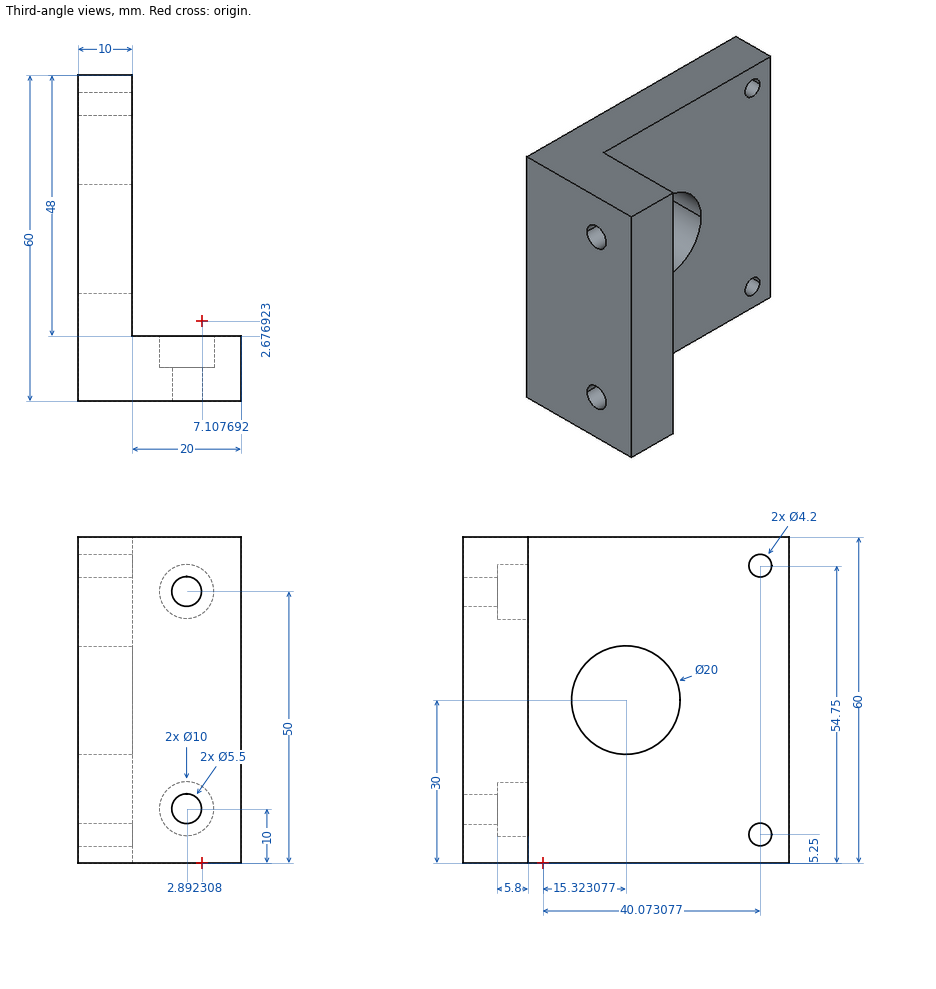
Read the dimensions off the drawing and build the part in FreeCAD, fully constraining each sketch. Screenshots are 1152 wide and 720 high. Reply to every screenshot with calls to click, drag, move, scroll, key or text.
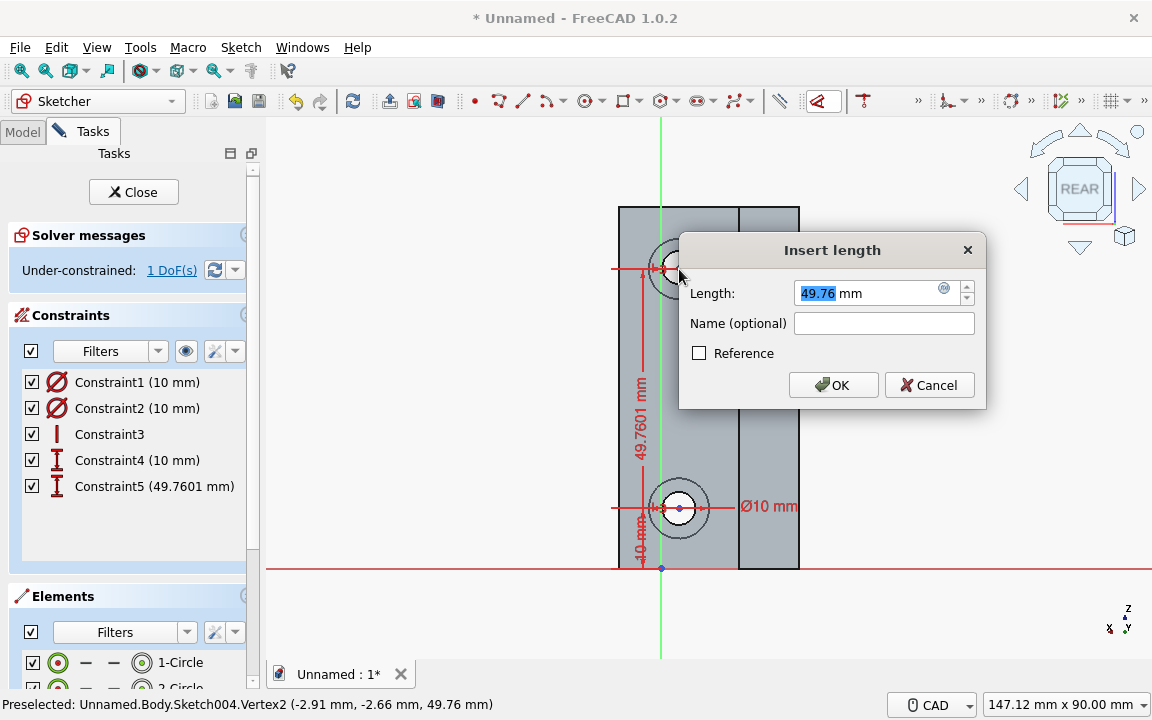
text(50)
key(Return)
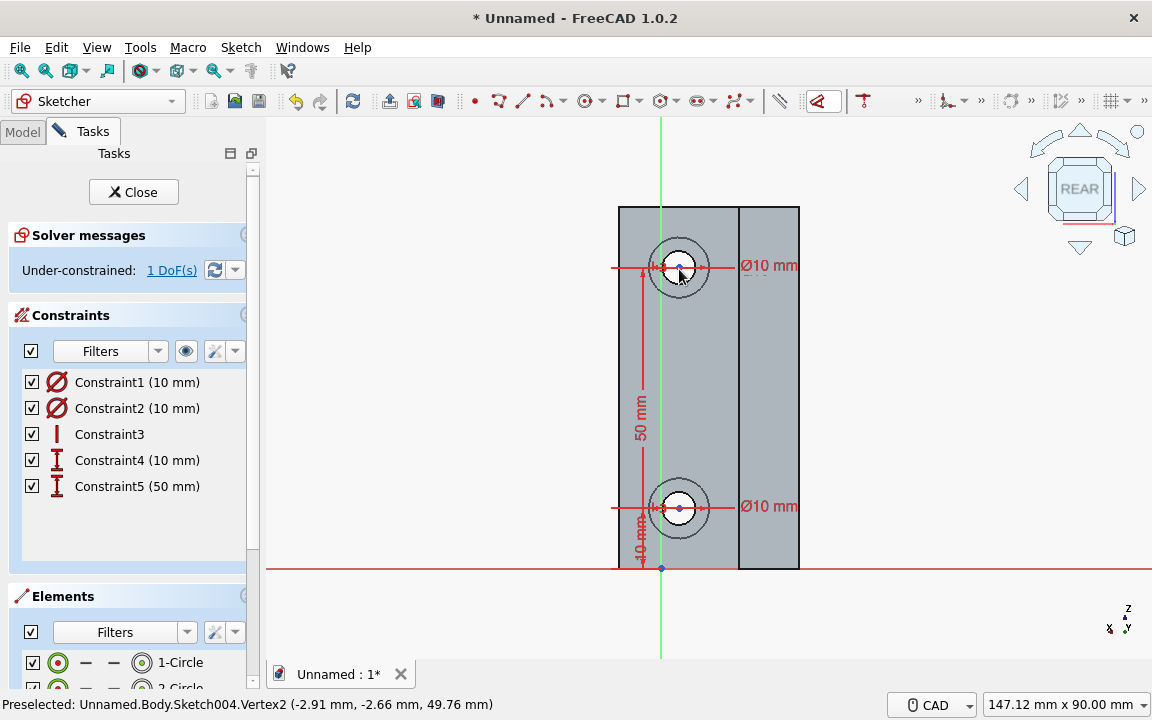
scroll(679, 508, up, 5)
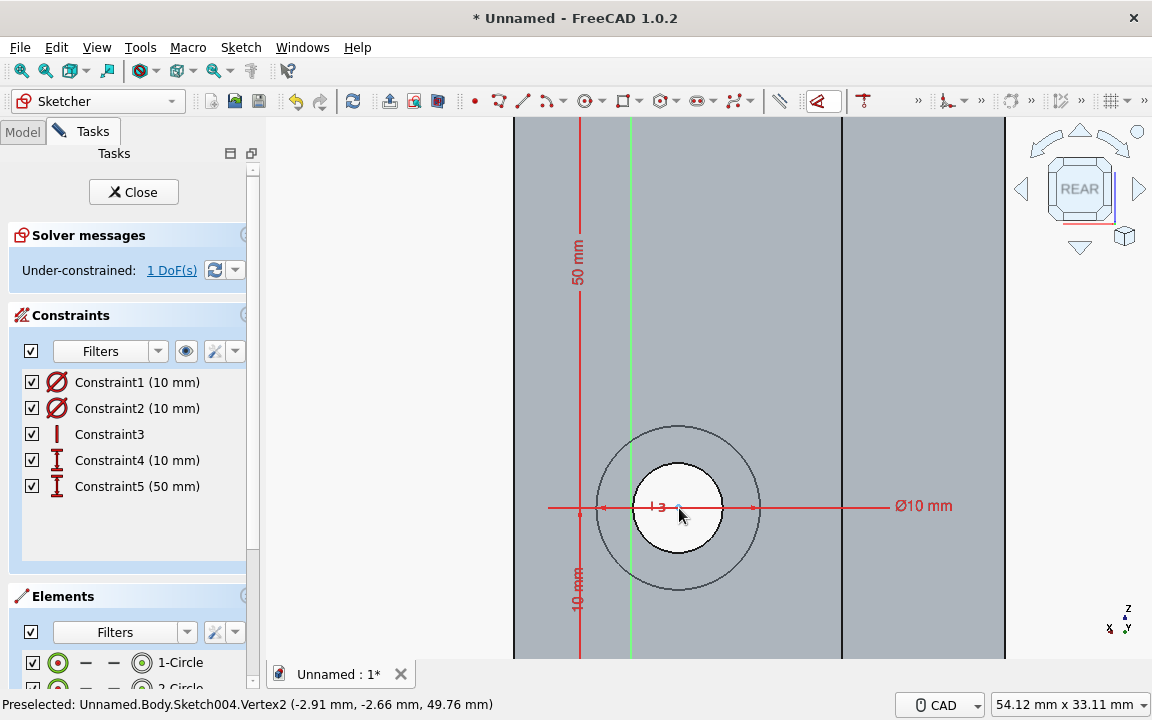
click(678, 508)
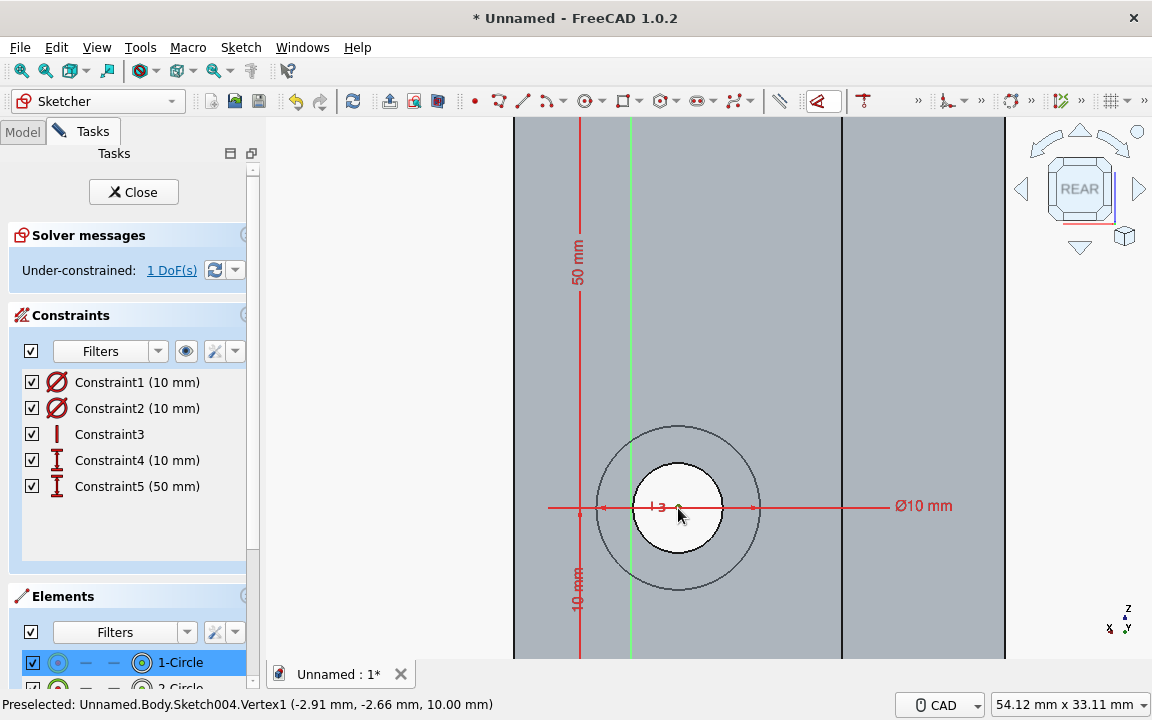
key(l)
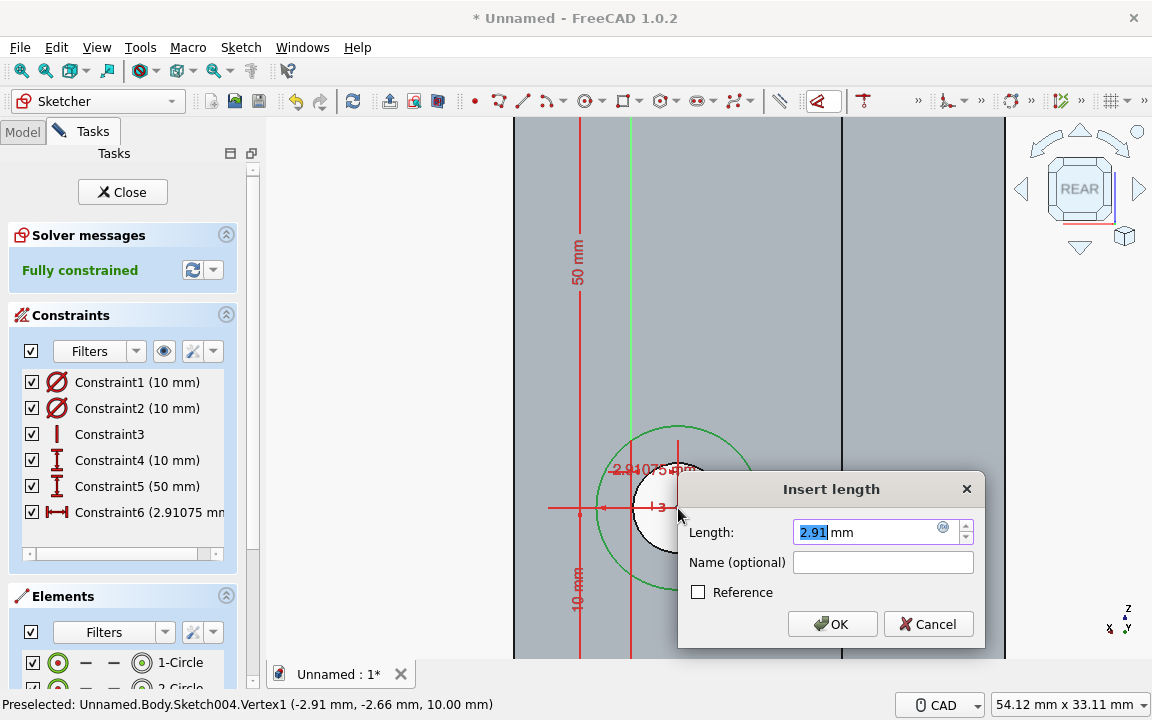
text(2.892308)
key(Return)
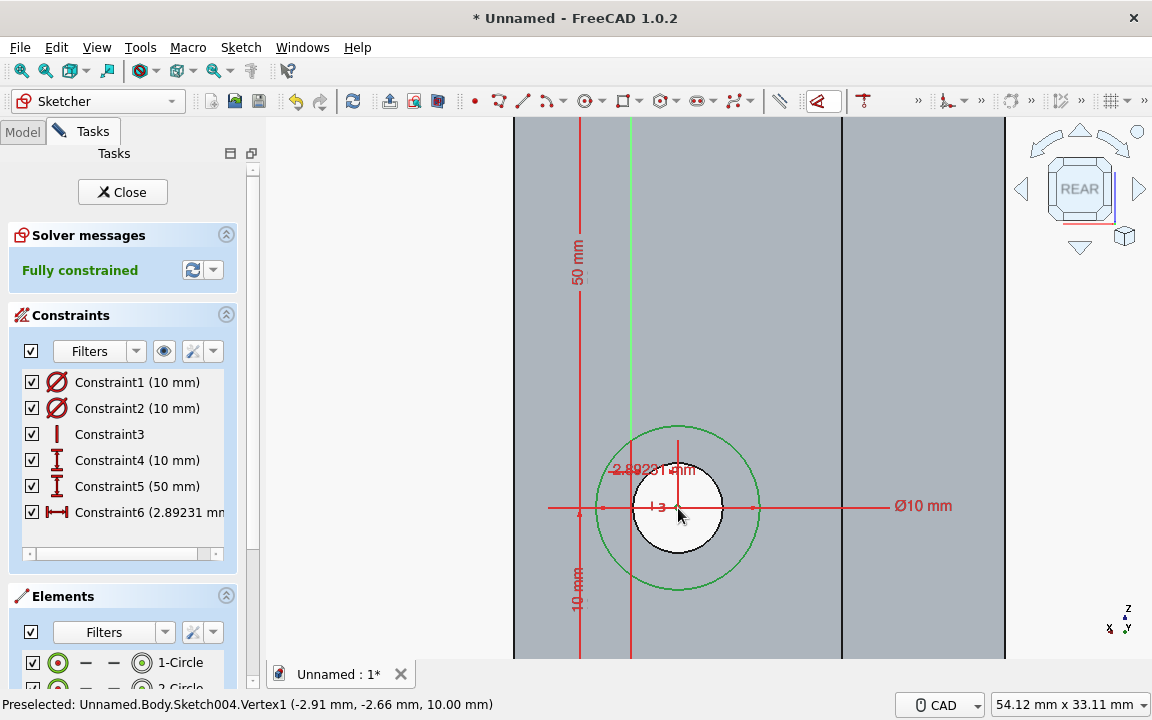
click(123, 192)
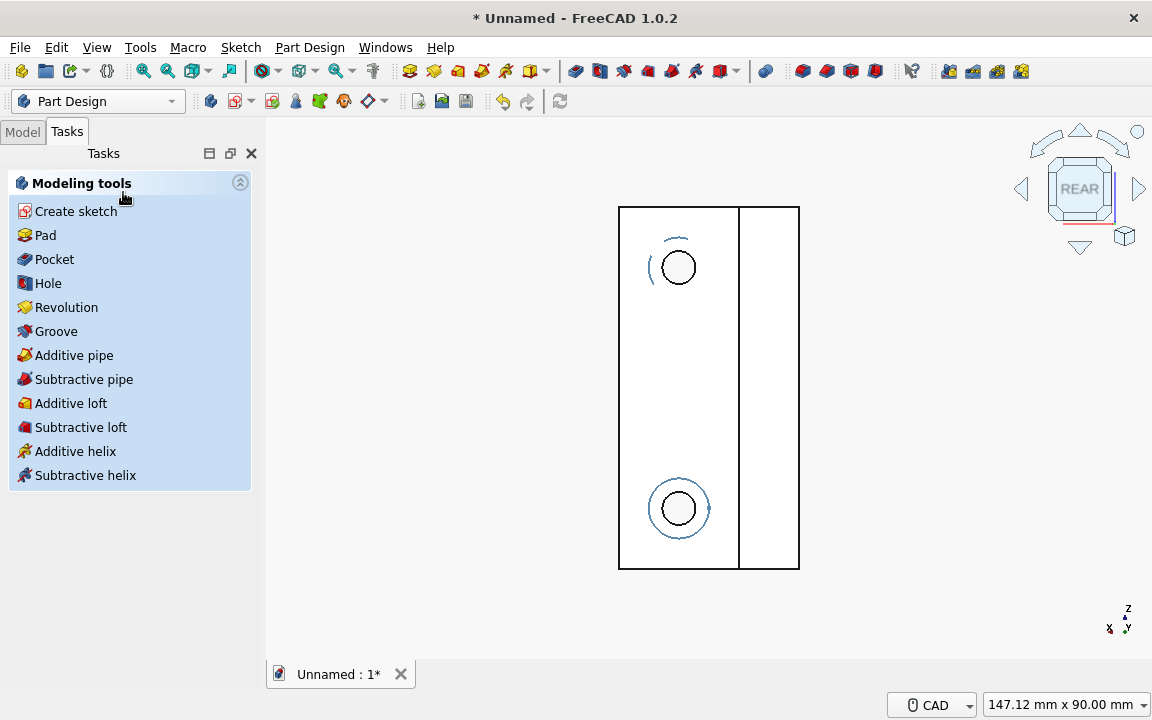
click(576, 72)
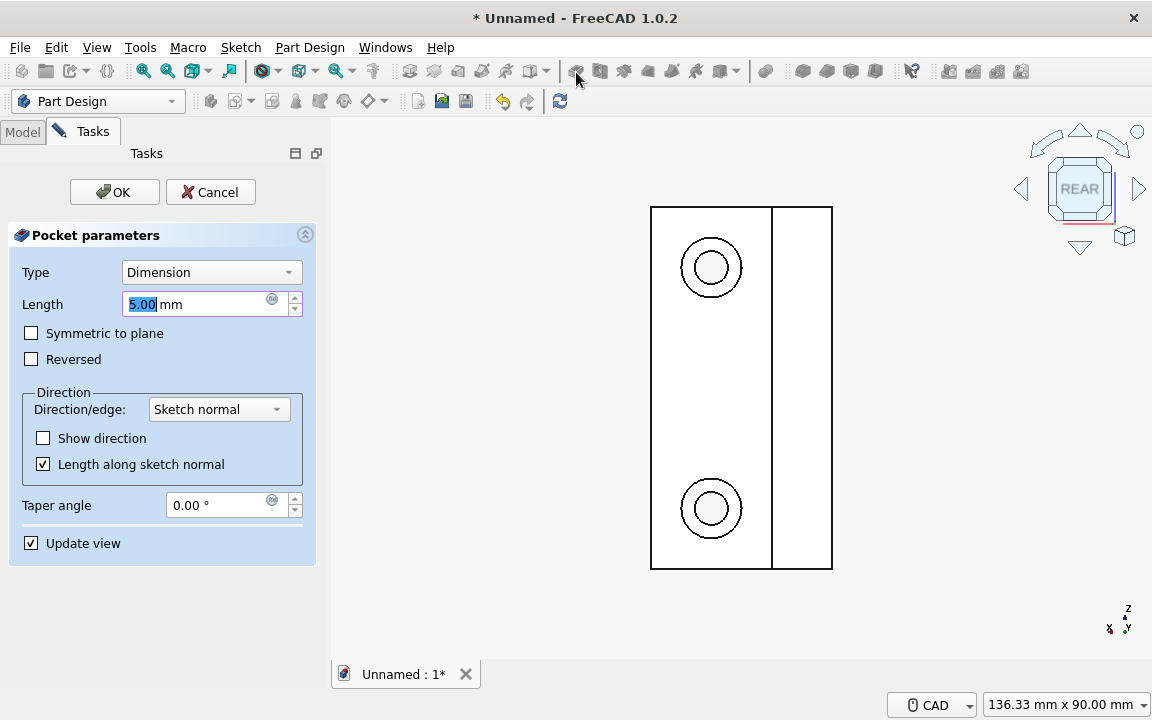
text(5.8)
key(Tab)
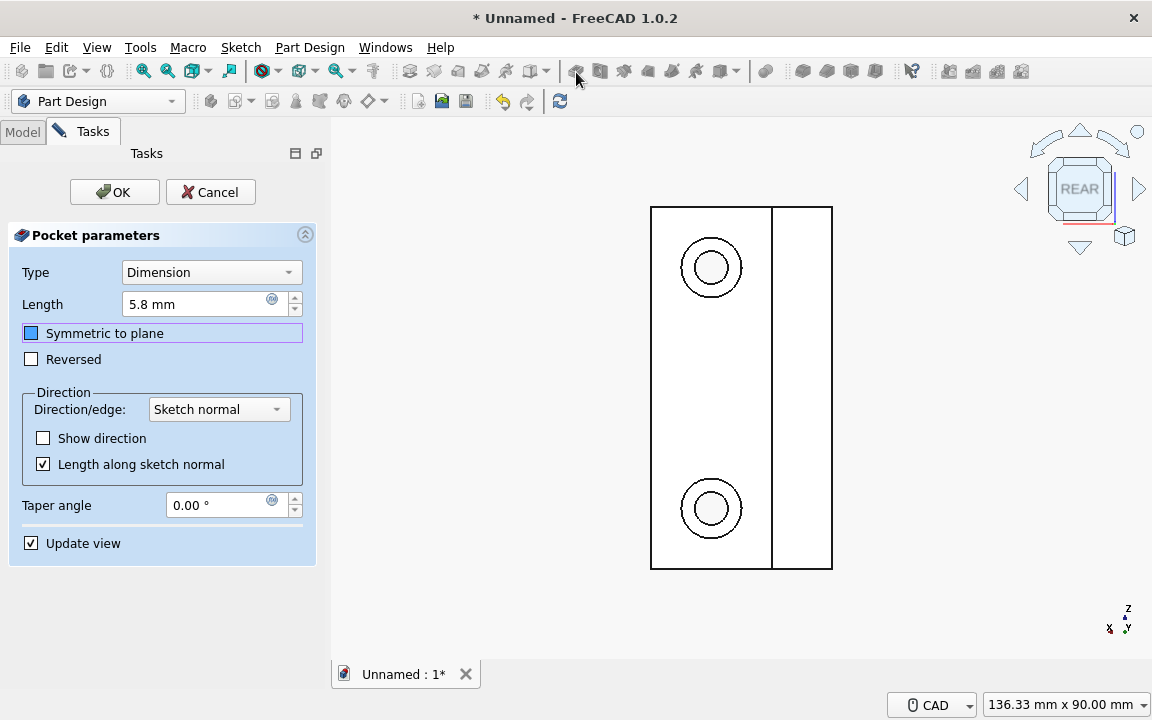
click(115, 192)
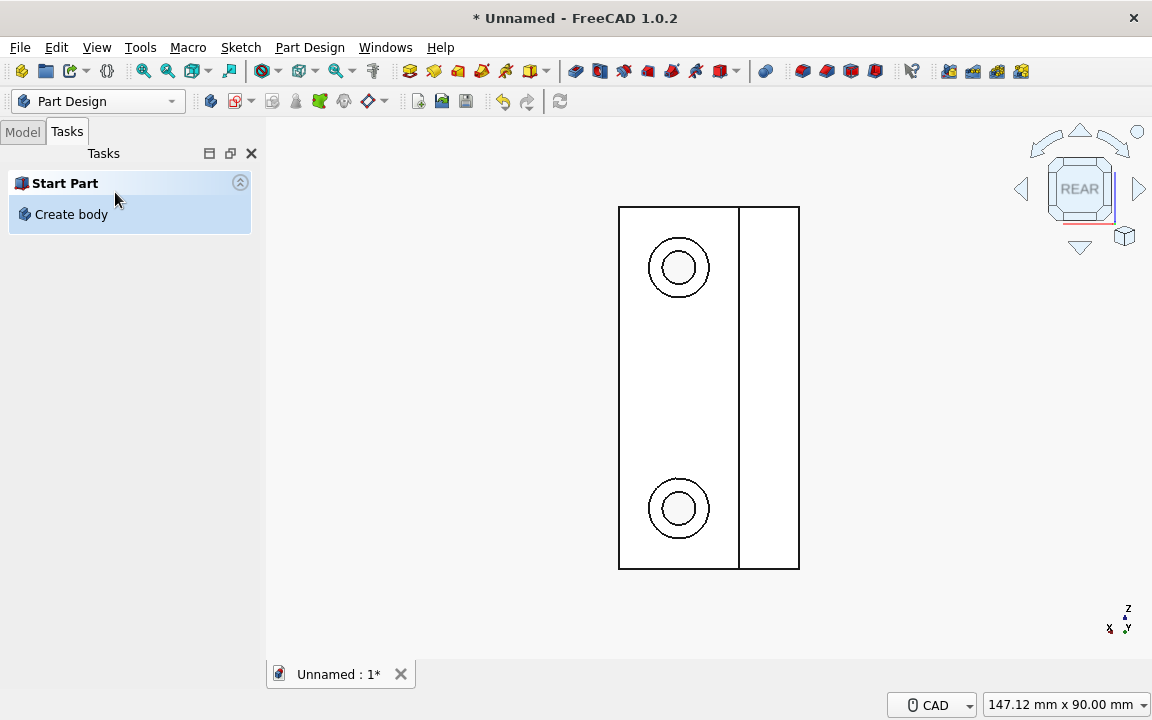
key(0)